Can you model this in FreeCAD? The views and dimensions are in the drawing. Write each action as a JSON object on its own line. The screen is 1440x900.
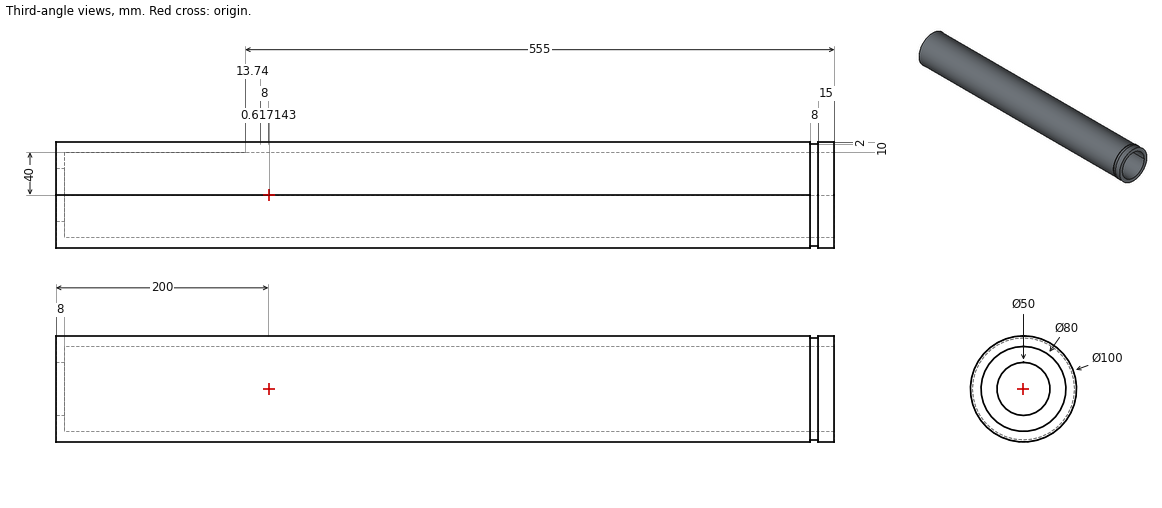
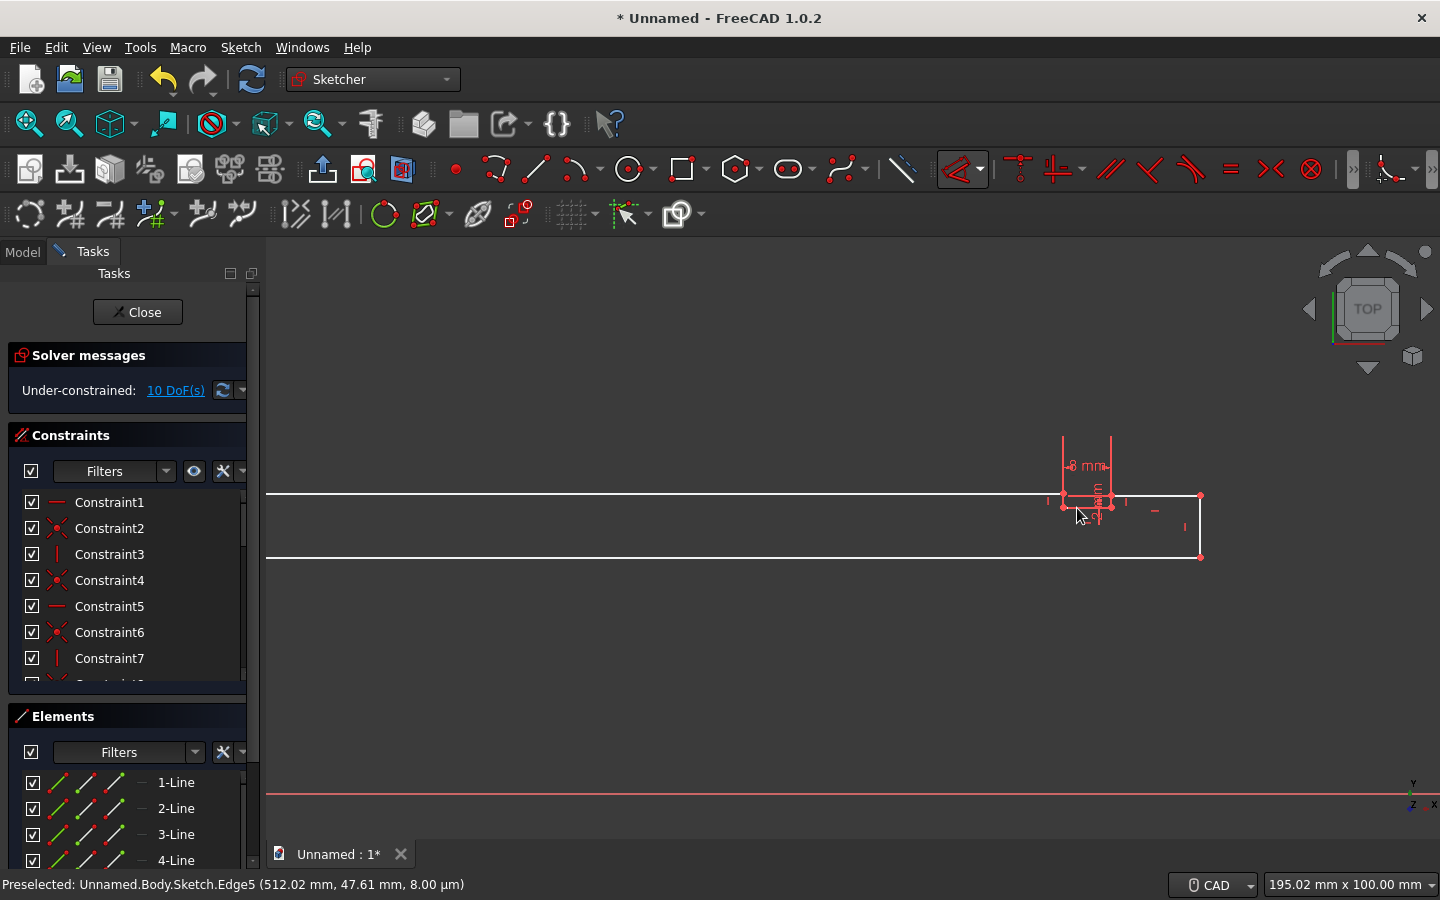
{"action": "scroll", "coordinate": [1063, 501], "scroll_direction": "up", "scroll_amount": 6}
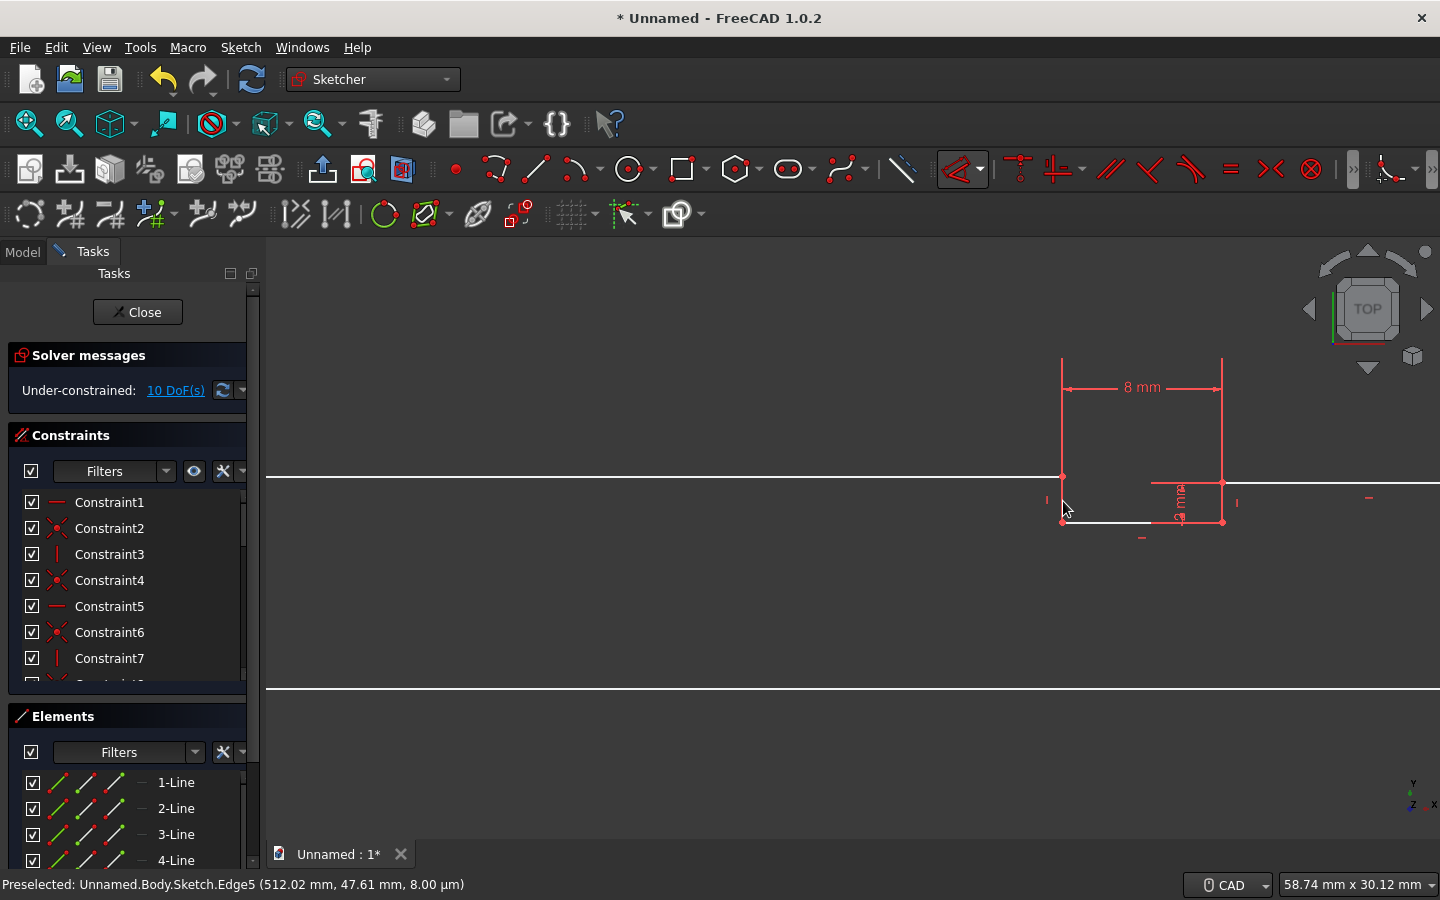
{"action": "left_click", "coordinate": [1062, 500]}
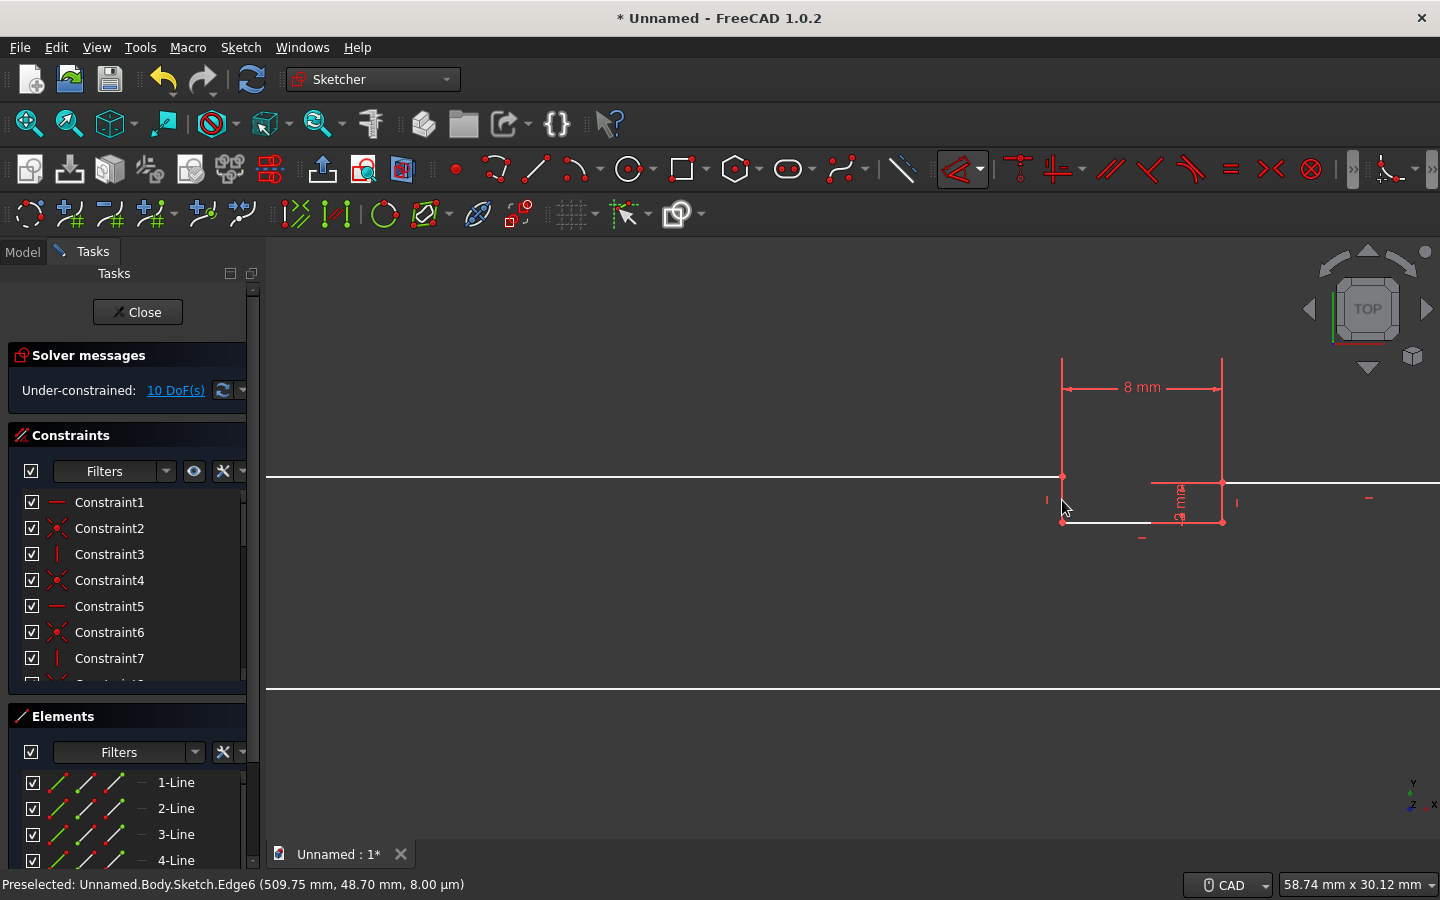
{"action": "key", "text": "i"}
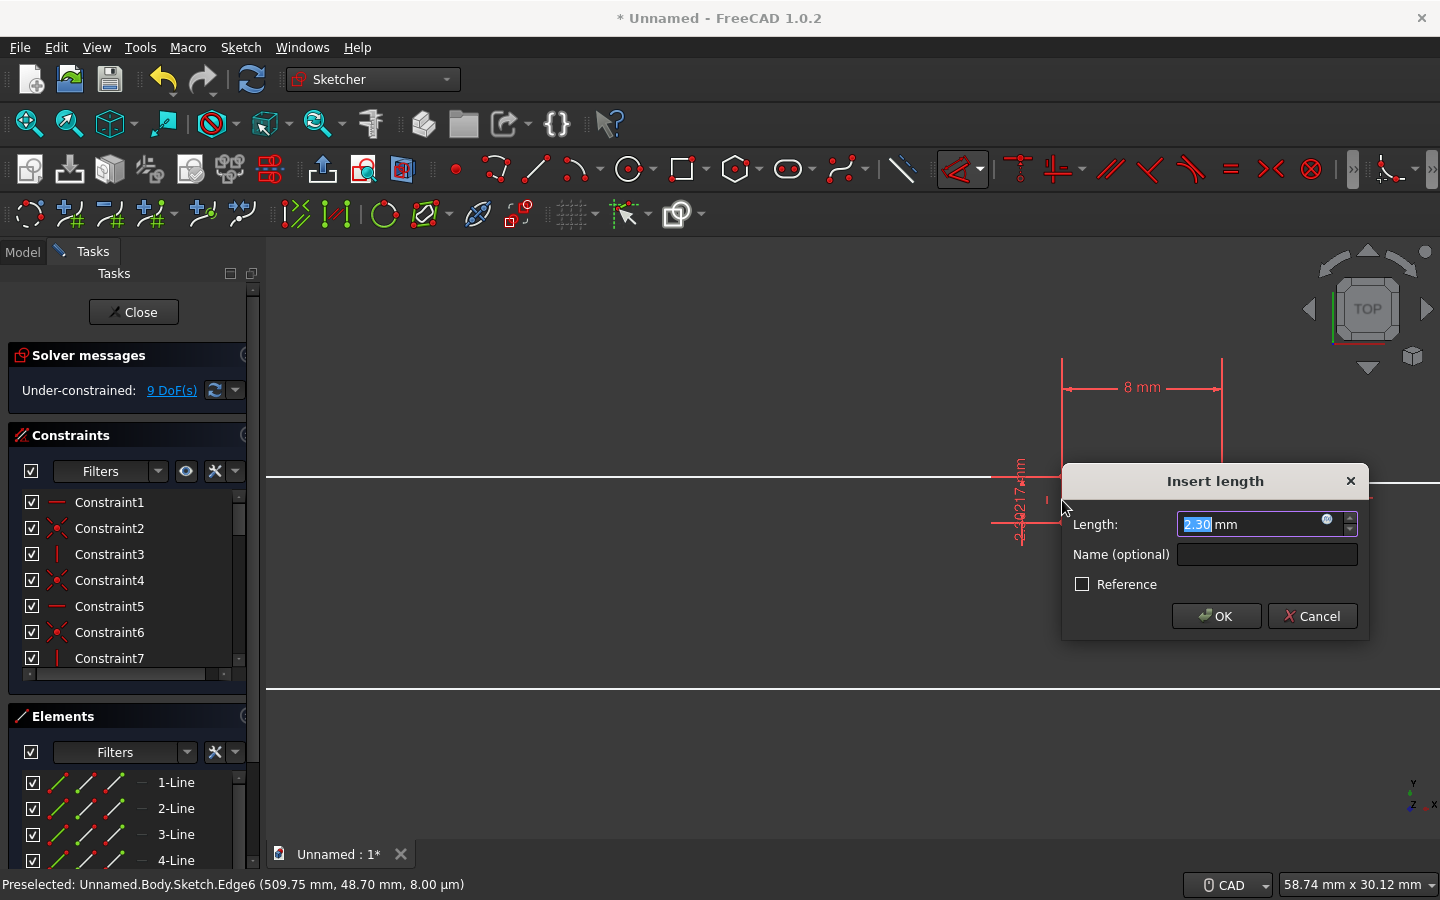
{"action": "type", "text": "2"}
{"action": "key", "text": "Return"}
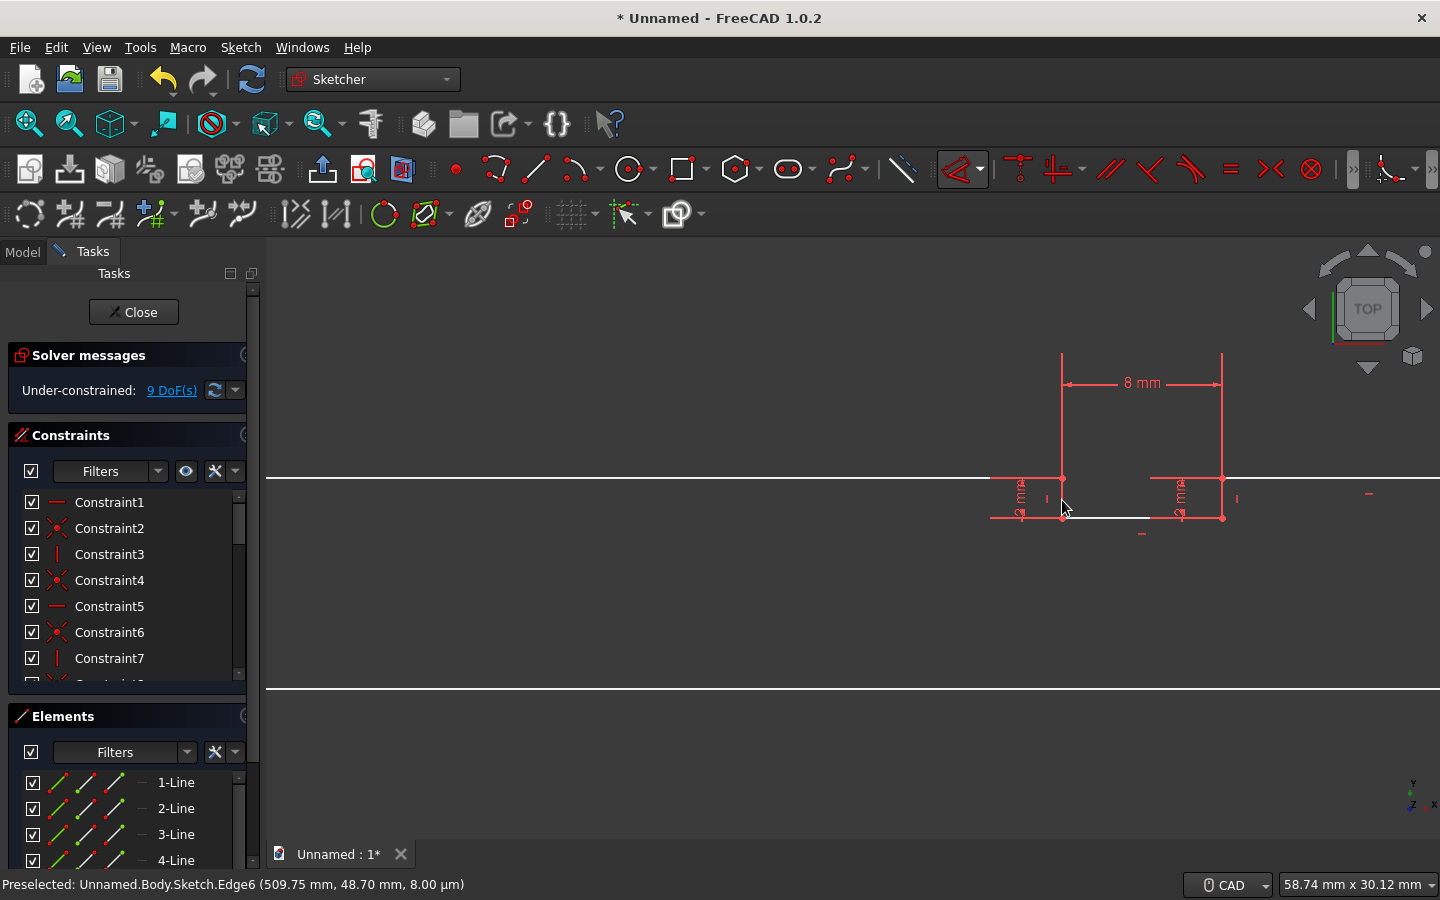
{"action": "scroll", "coordinate": [1096, 510], "scroll_direction": "down", "scroll_amount": 14}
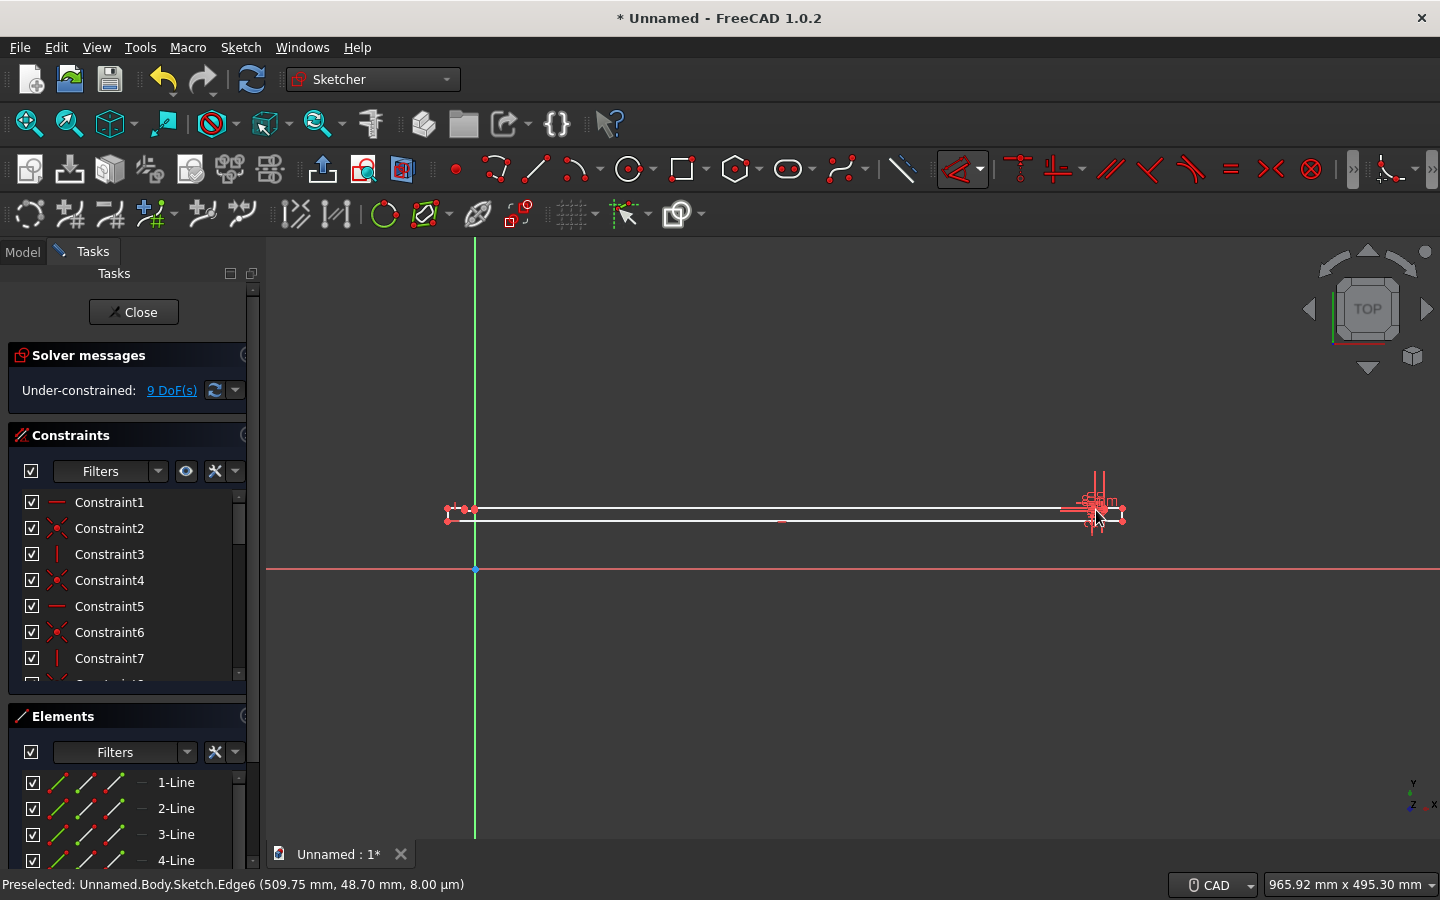
{"action": "scroll", "coordinate": [474, 509], "scroll_direction": "up", "scroll_amount": 14}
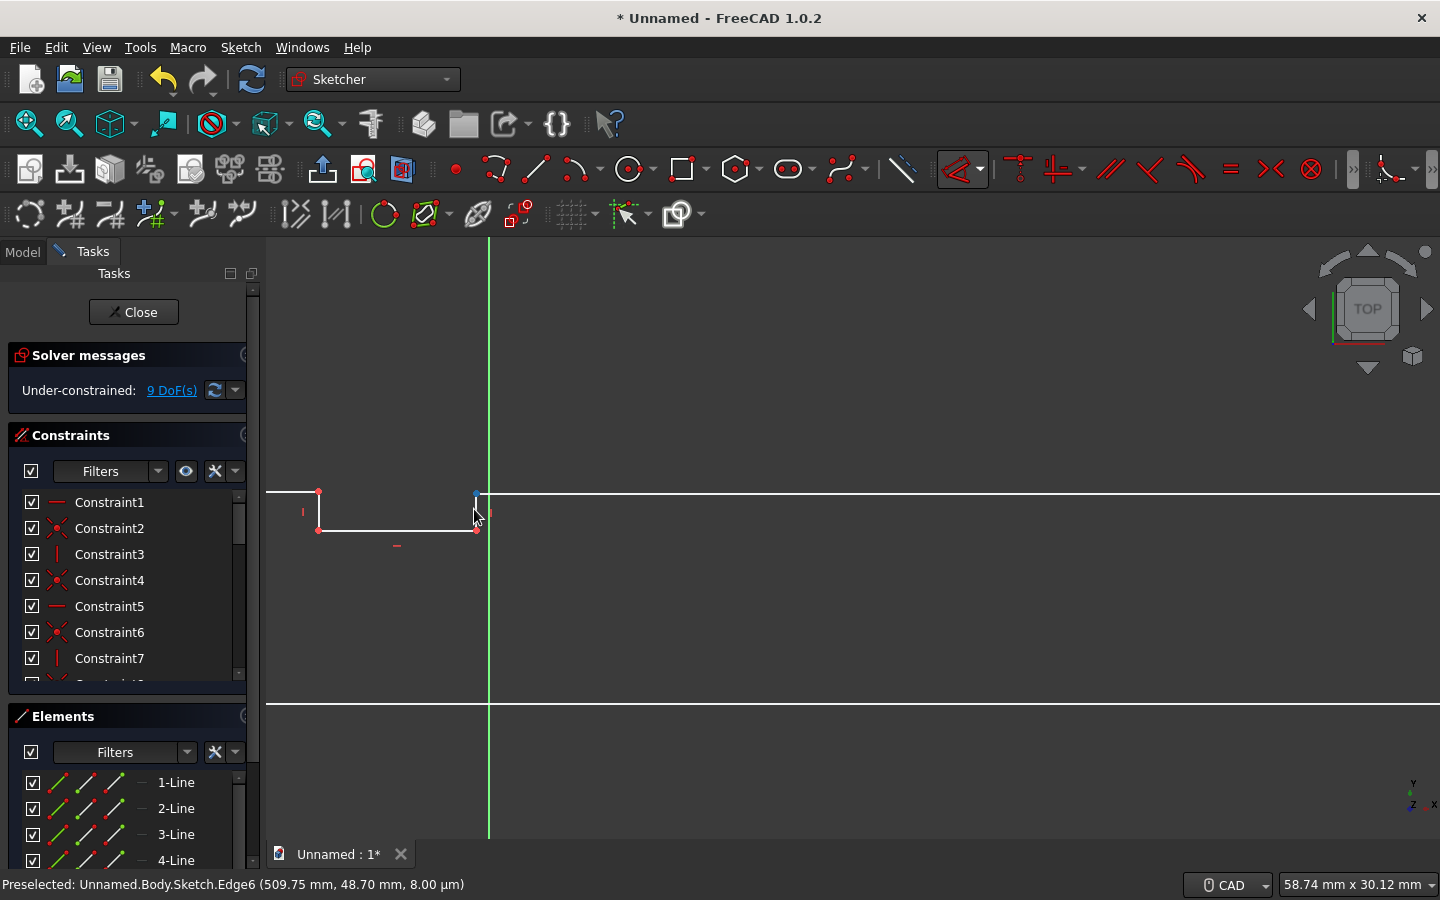
{"action": "left_click", "coordinate": [476, 505]}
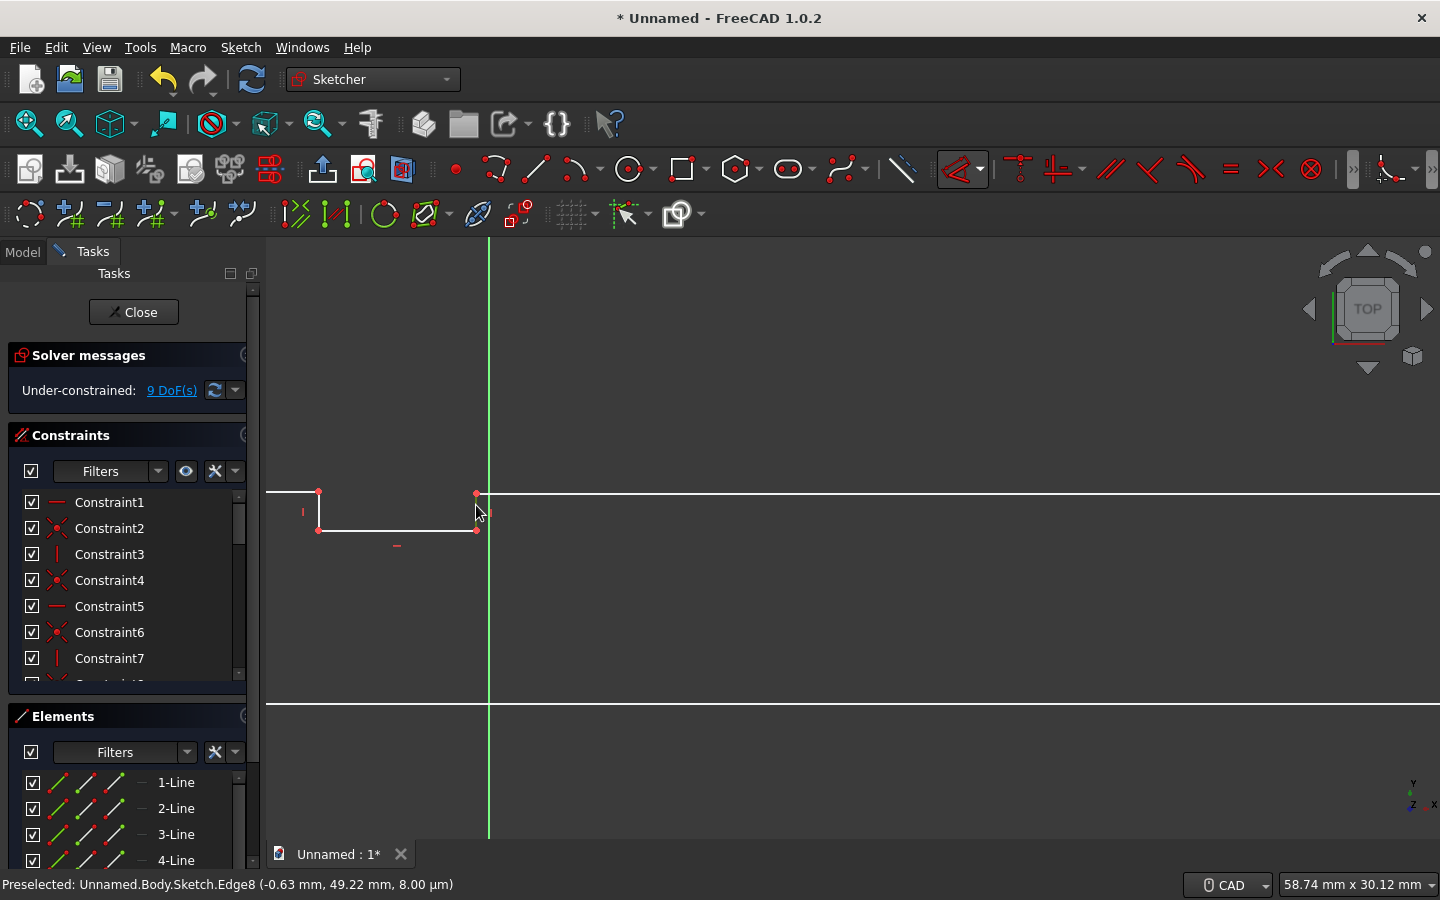
{"action": "key", "text": "i"}